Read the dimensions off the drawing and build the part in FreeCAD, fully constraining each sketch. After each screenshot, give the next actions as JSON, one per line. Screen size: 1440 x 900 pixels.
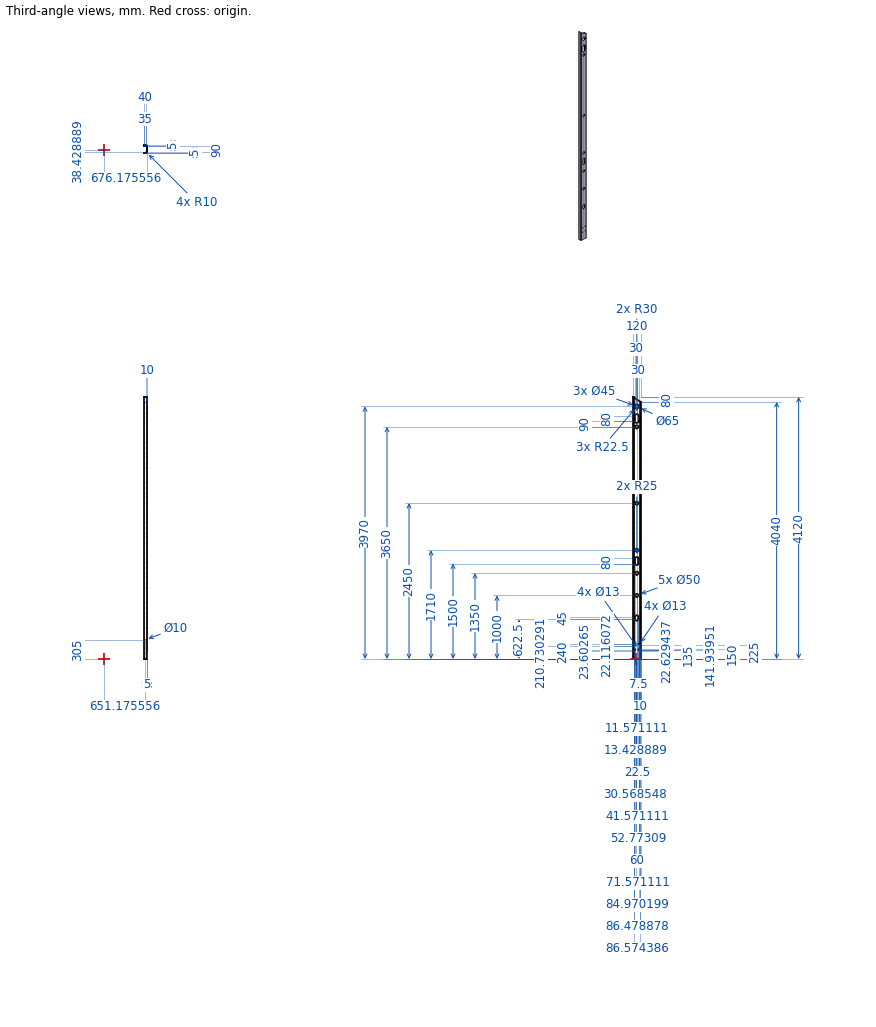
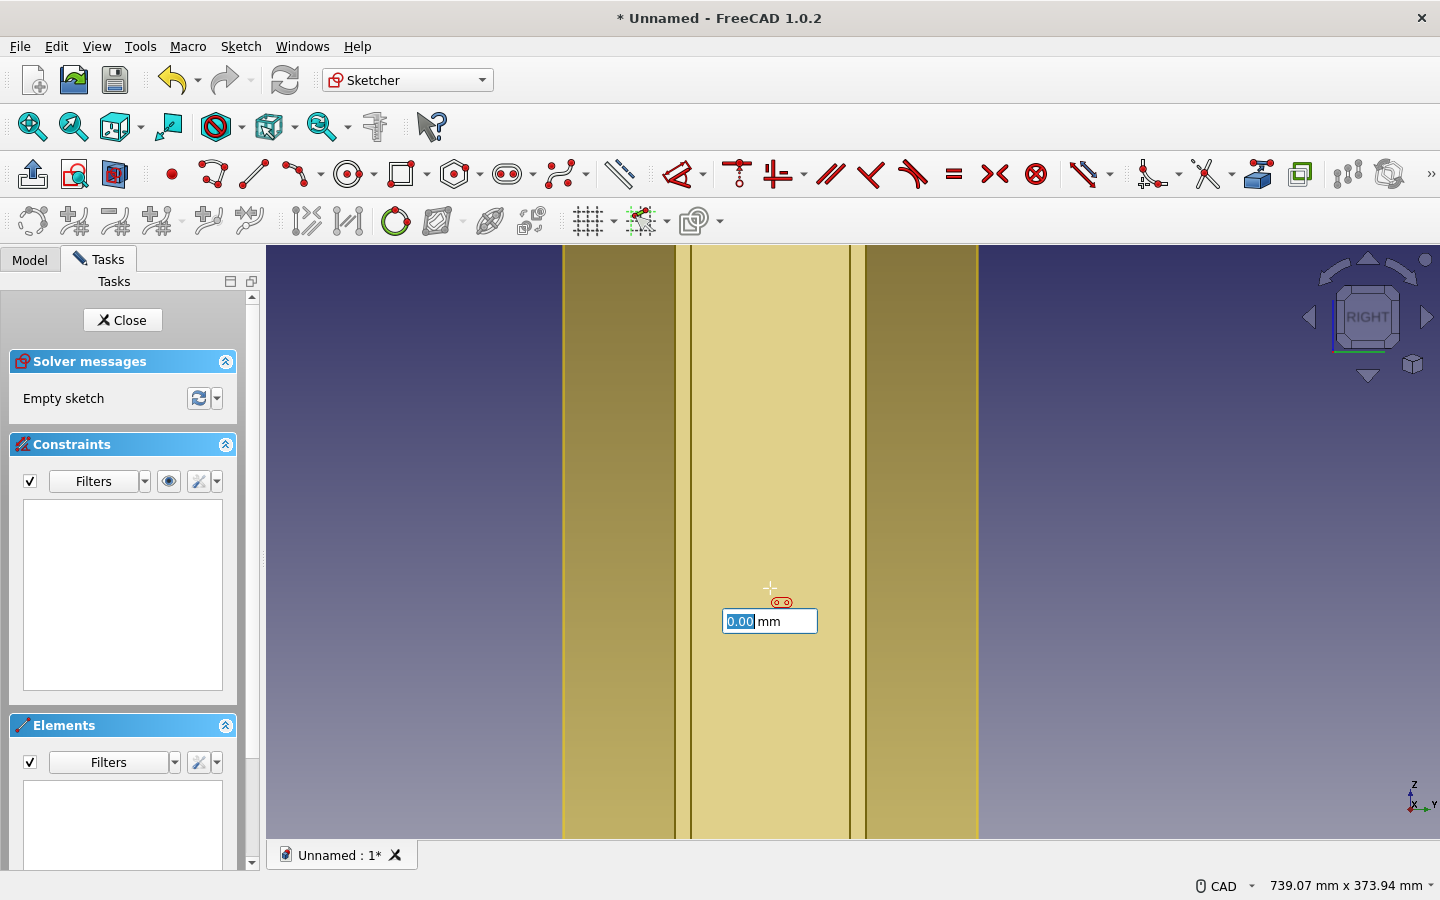
{"action": "left_click", "coordinate": [806, 624]}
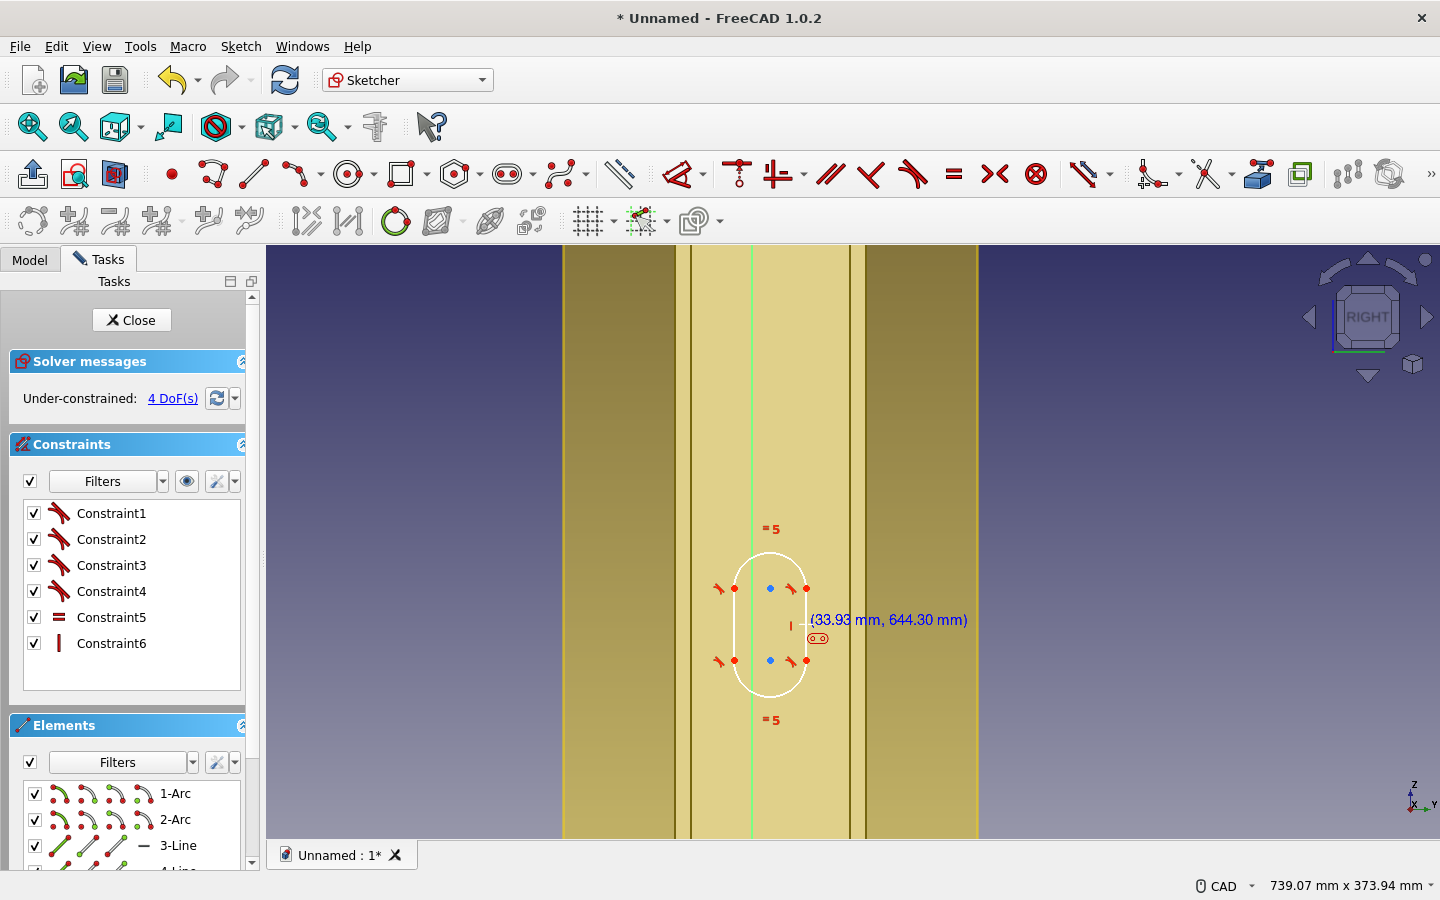
{"action": "scroll", "coordinate": [785, 676], "scroll_direction": "down", "scroll_amount": 14}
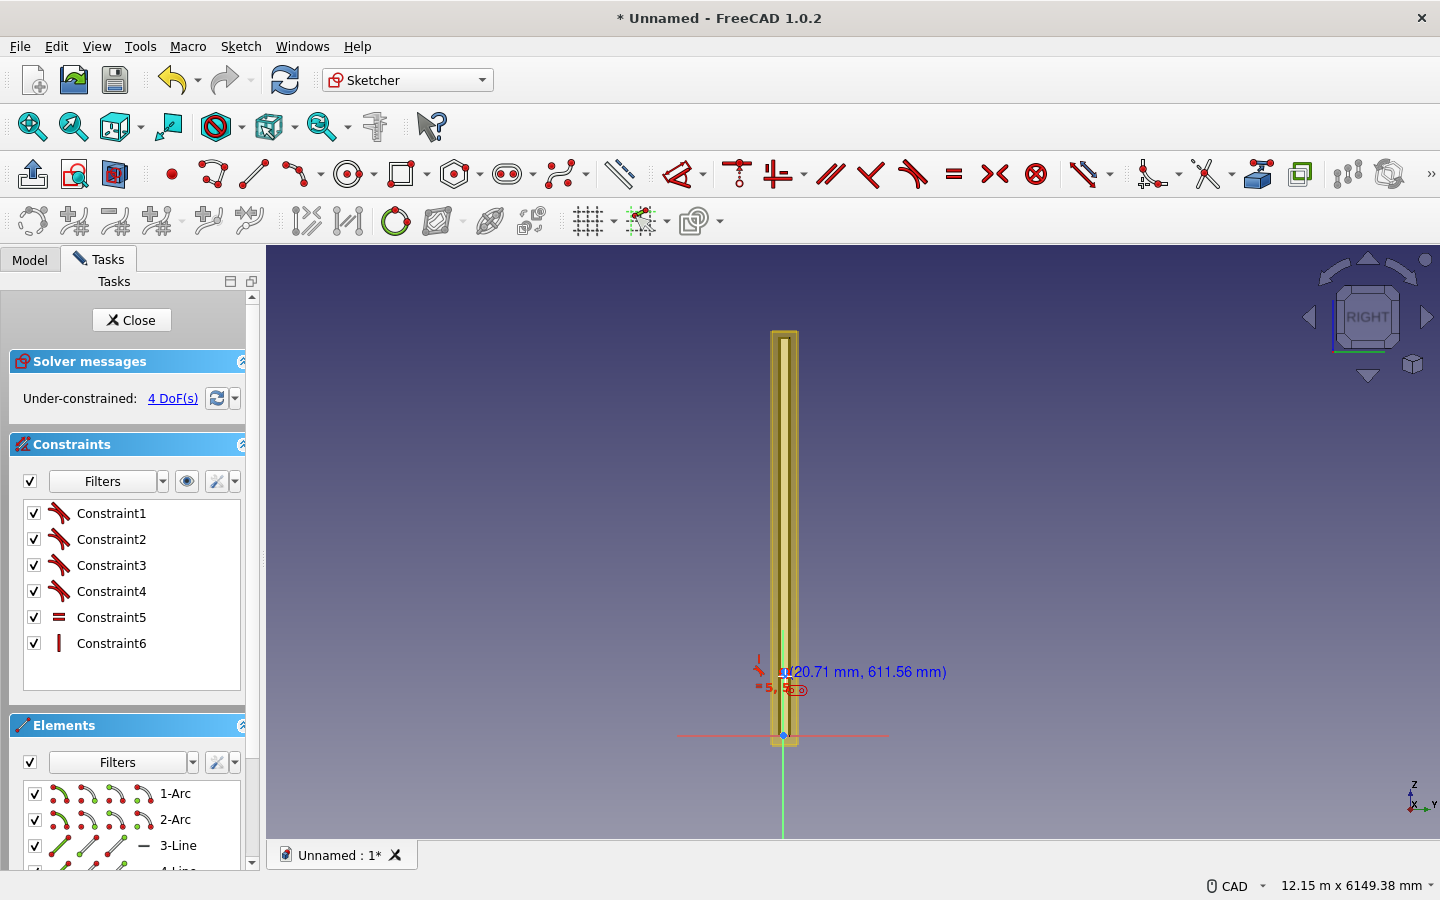
{"action": "scroll", "coordinate": [785, 375], "scroll_direction": "up", "scroll_amount": 14}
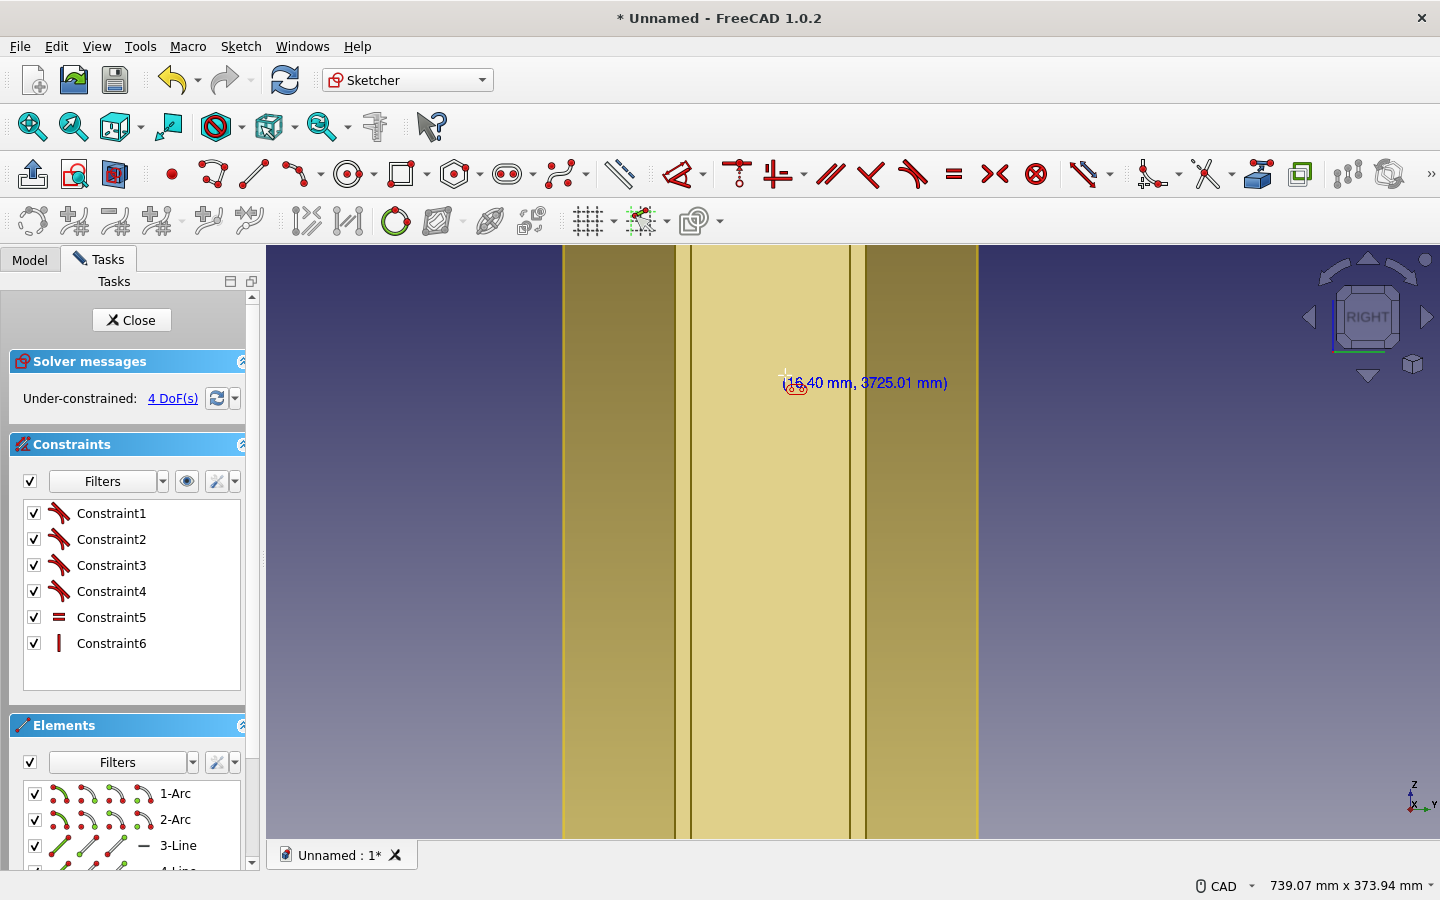
{"action": "left_click", "coordinate": [770, 364]}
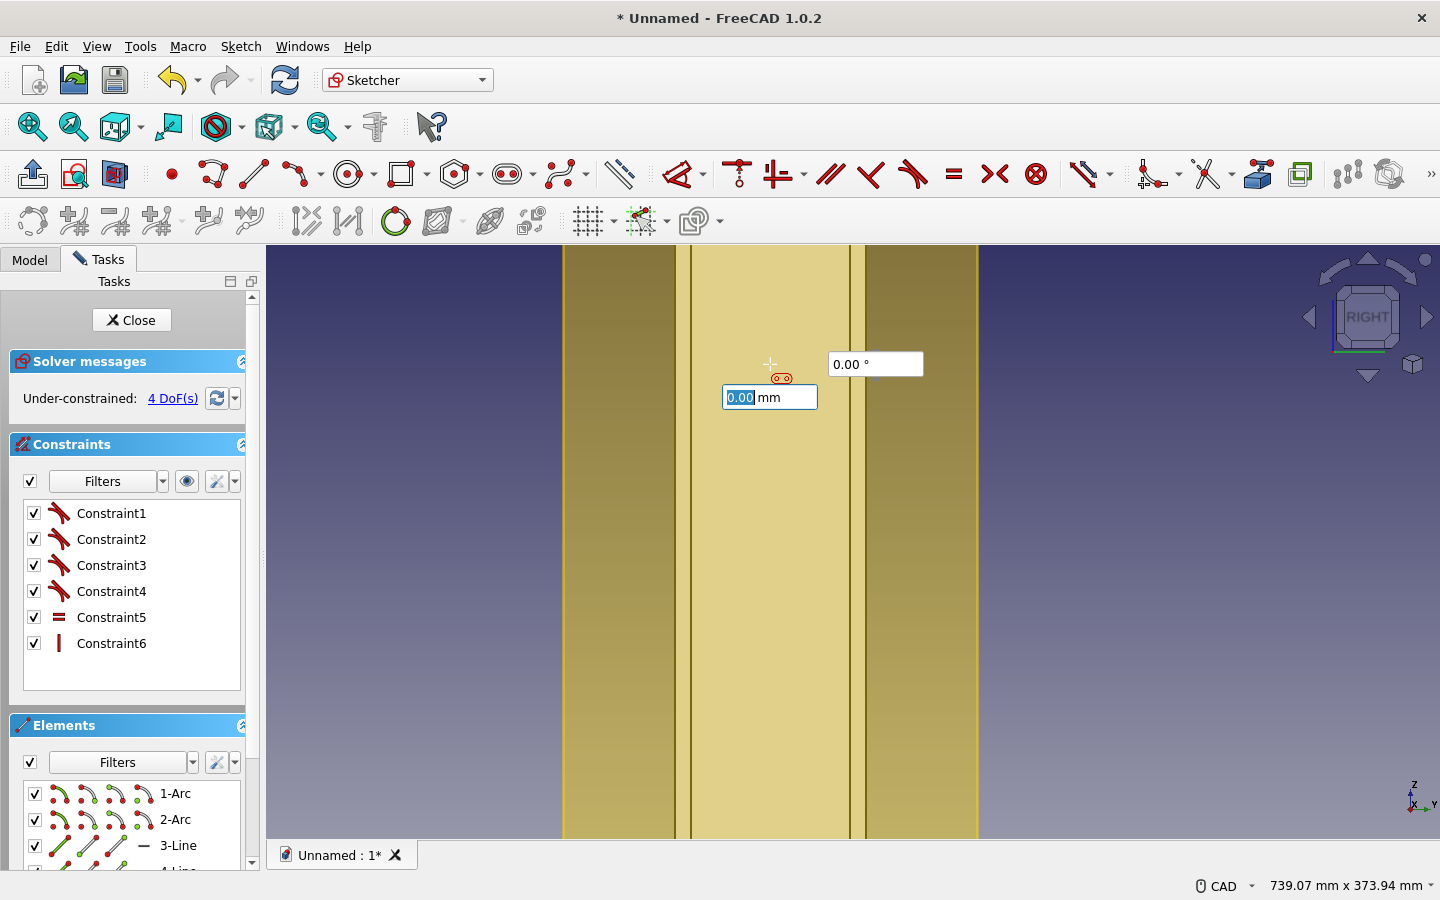
{"action": "scroll", "coordinate": [785, 374], "scroll_direction": "down", "scroll_amount": 14}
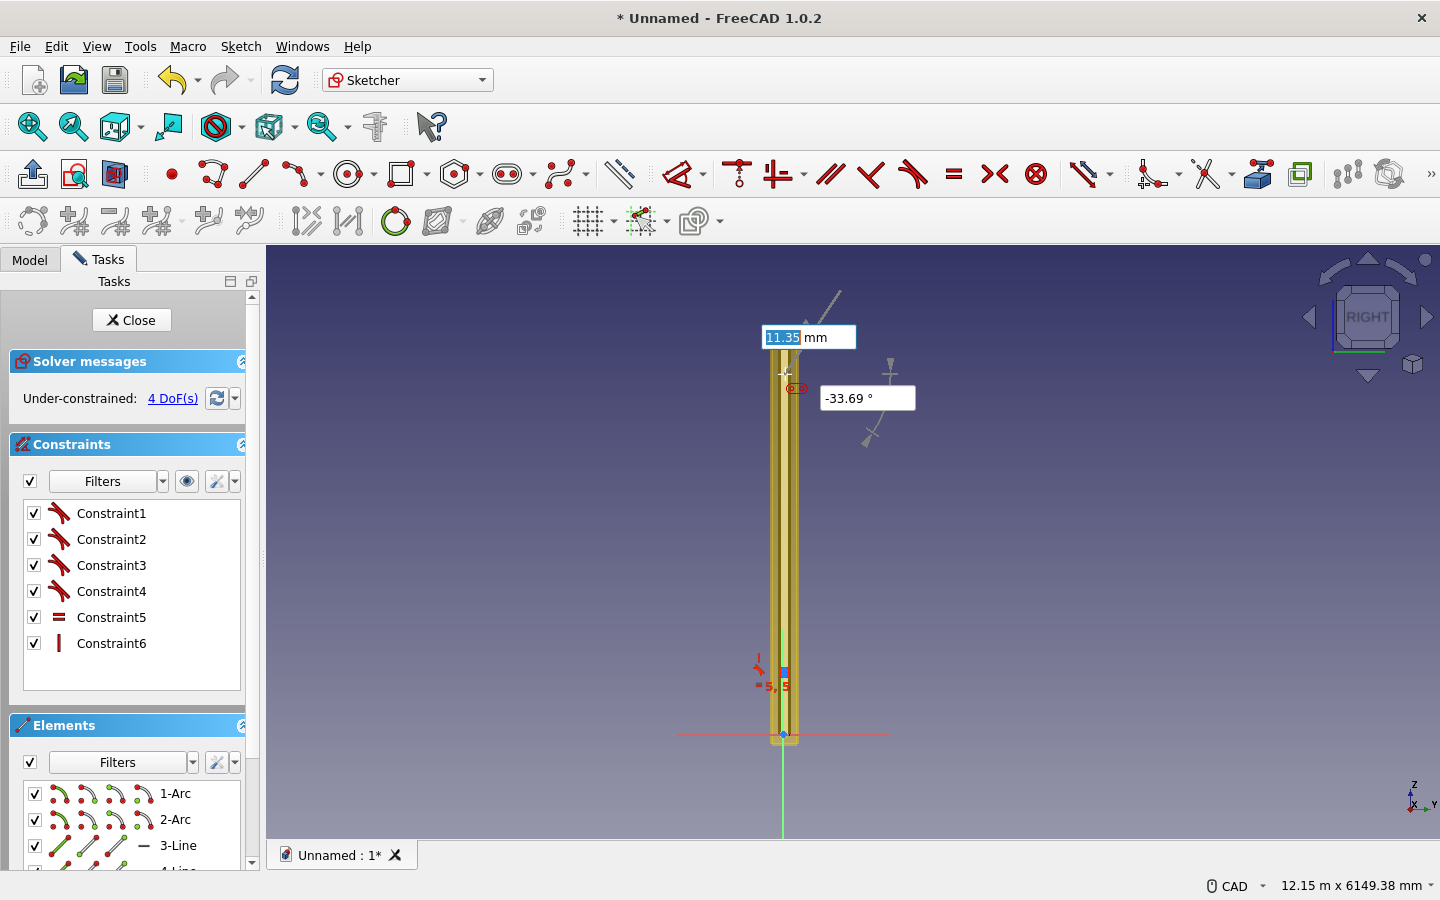
{"action": "scroll", "coordinate": [785, 366], "scroll_direction": "up", "scroll_amount": 14}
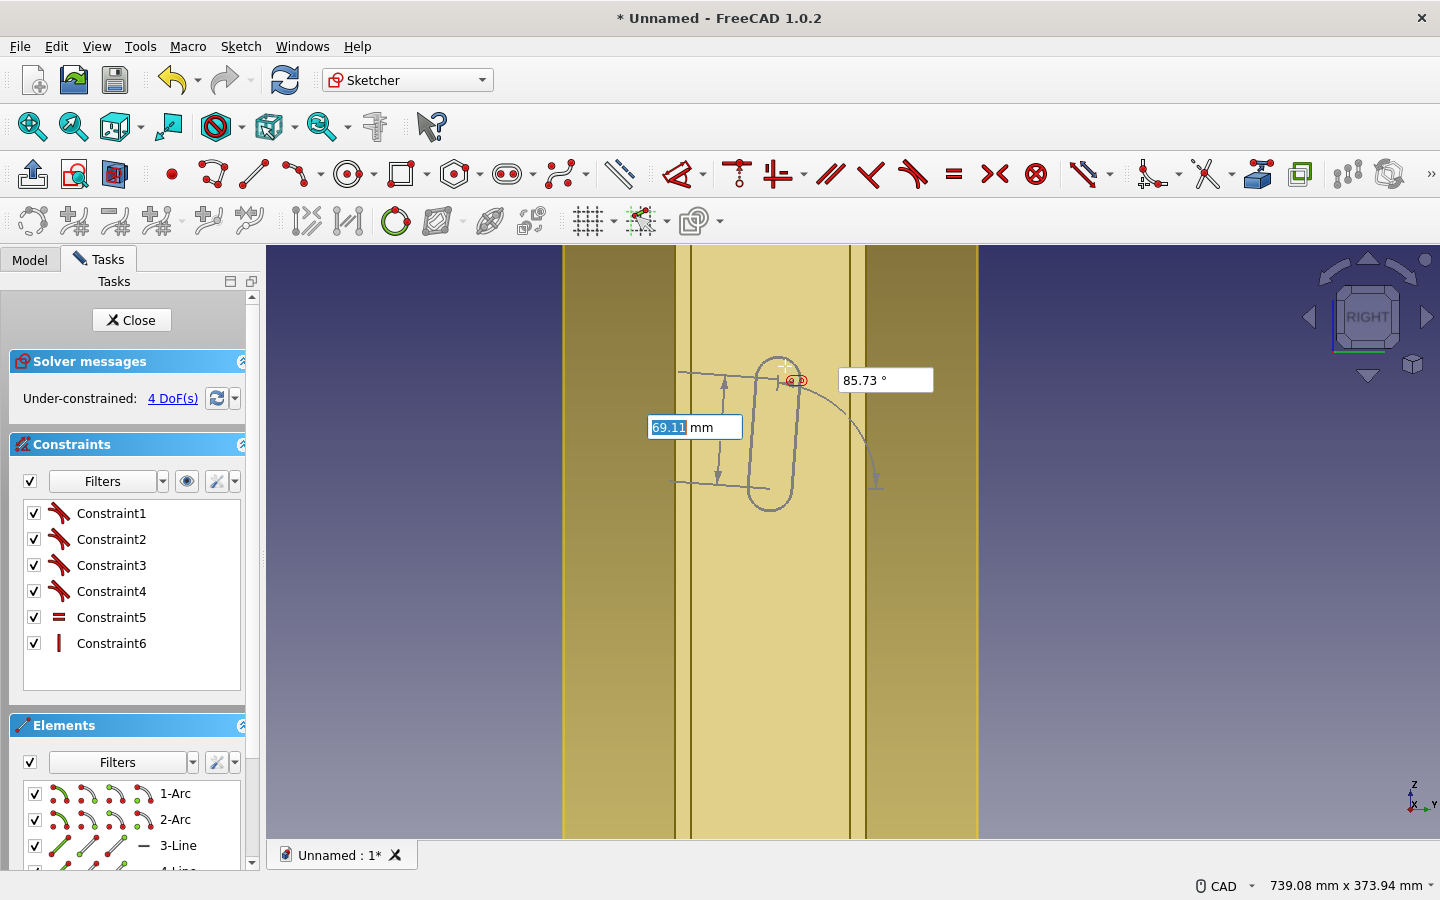
{"action": "left_click", "coordinate": [770, 361]}